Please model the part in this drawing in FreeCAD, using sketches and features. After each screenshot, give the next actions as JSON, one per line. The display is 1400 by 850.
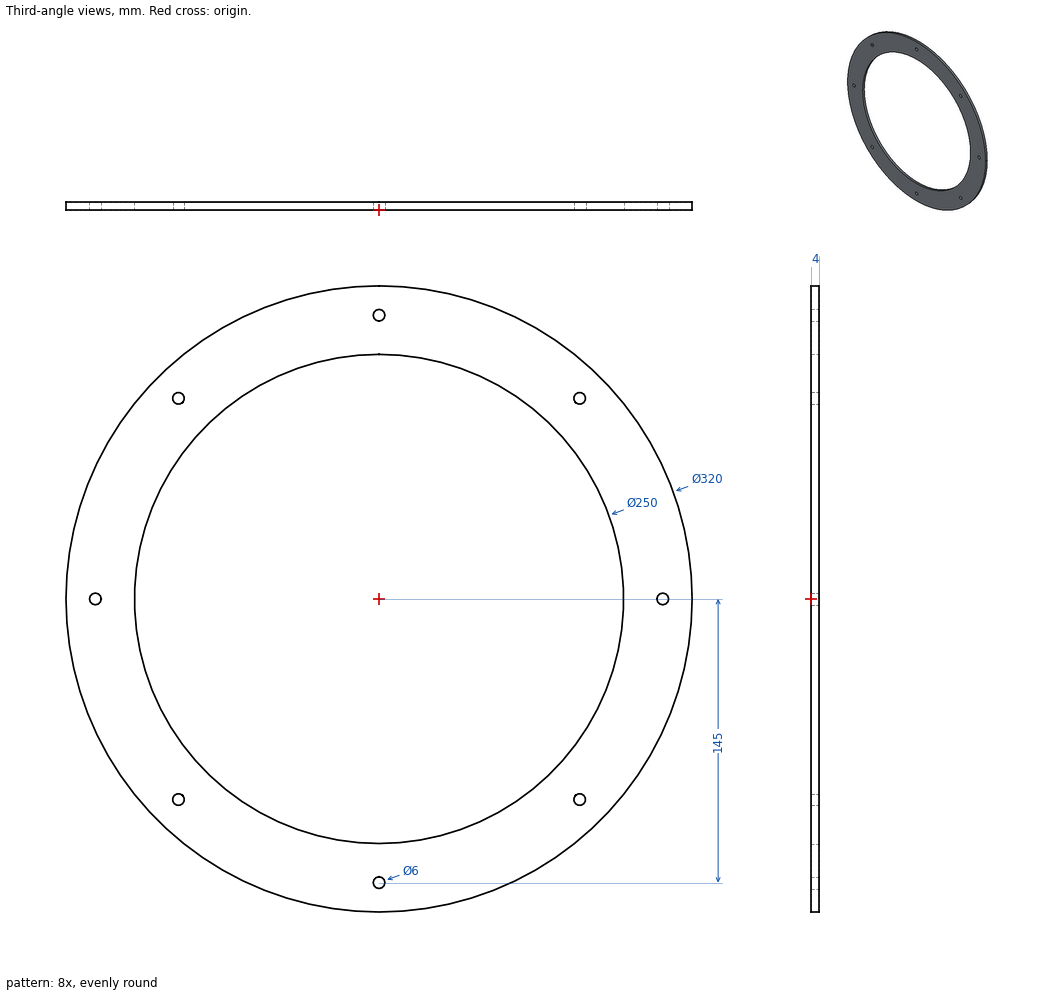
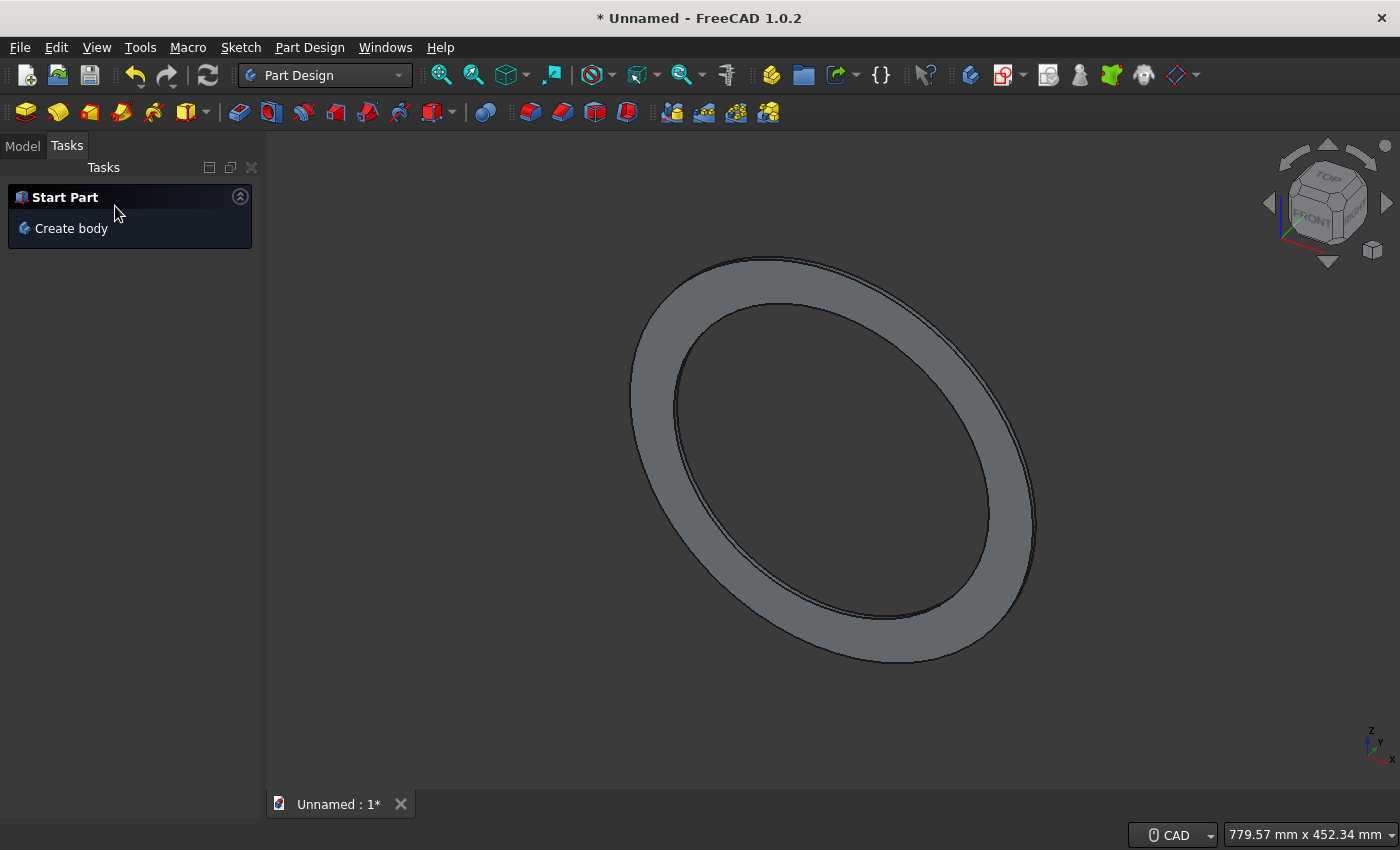
{"action": "key", "text": "4"}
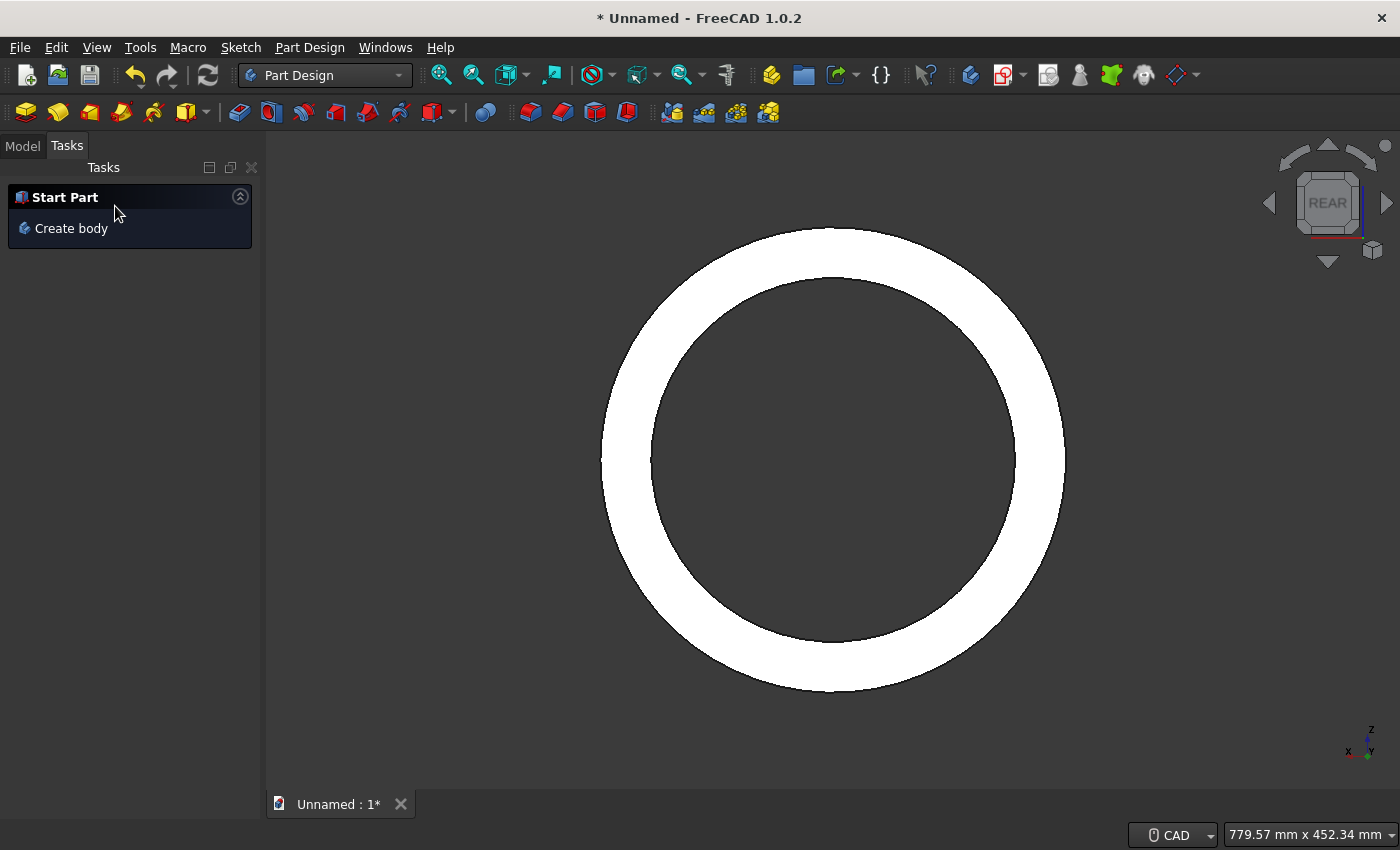
{"action": "left_click", "coordinate": [900, 658]}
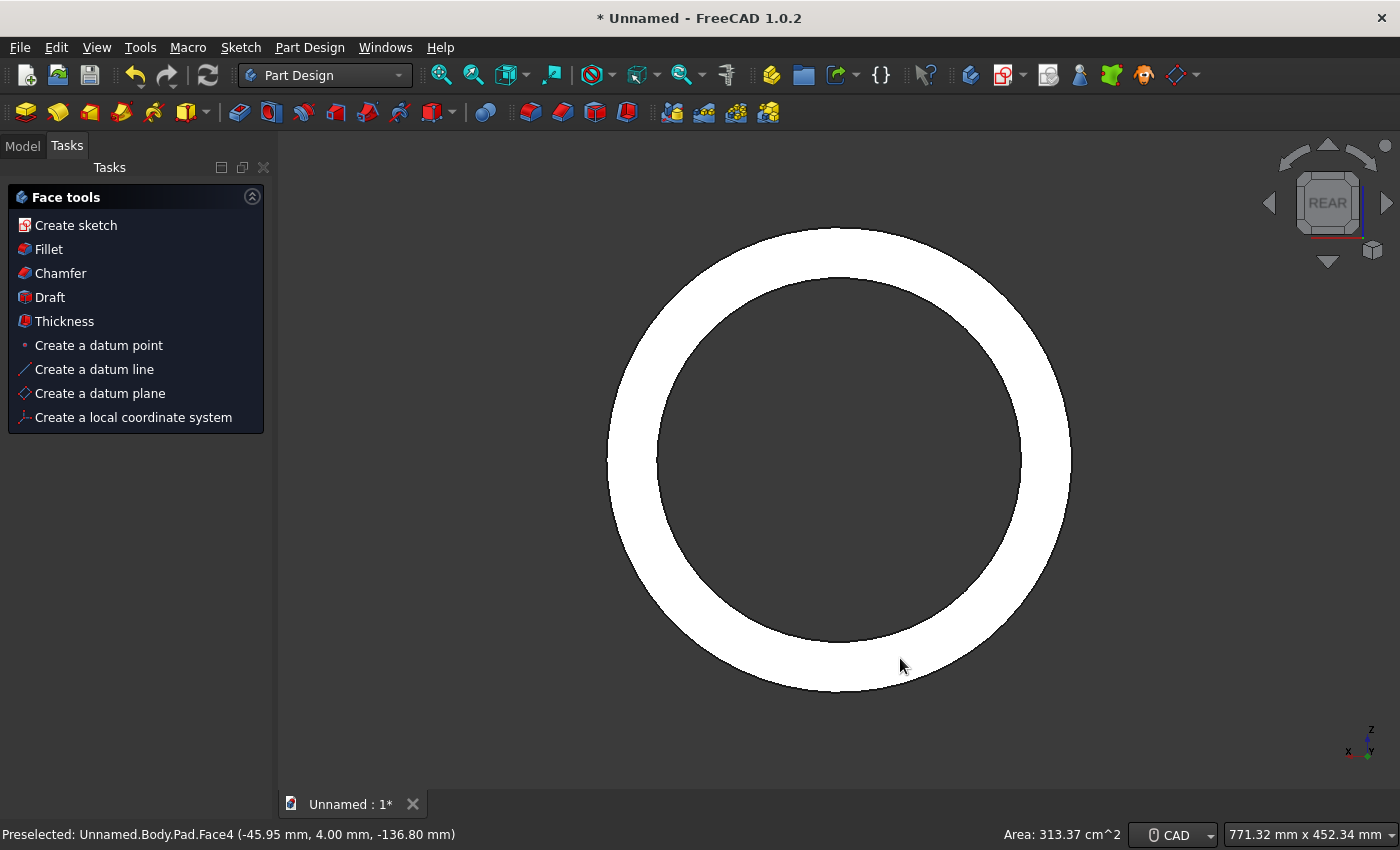
{"action": "left_click", "coordinate": [1004, 76]}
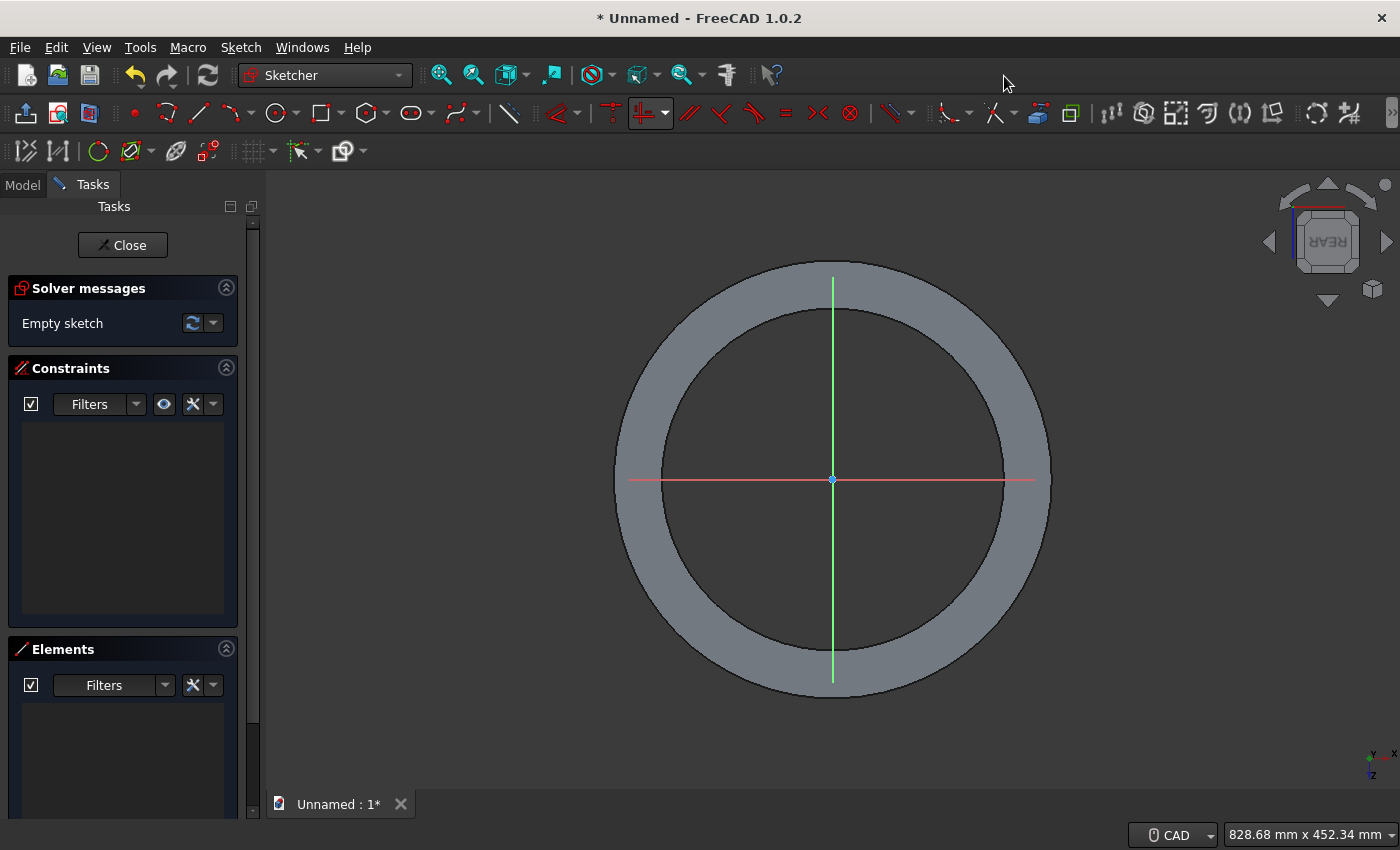
{"action": "scroll", "coordinate": [836, 271], "scroll_direction": "up", "scroll_amount": 15}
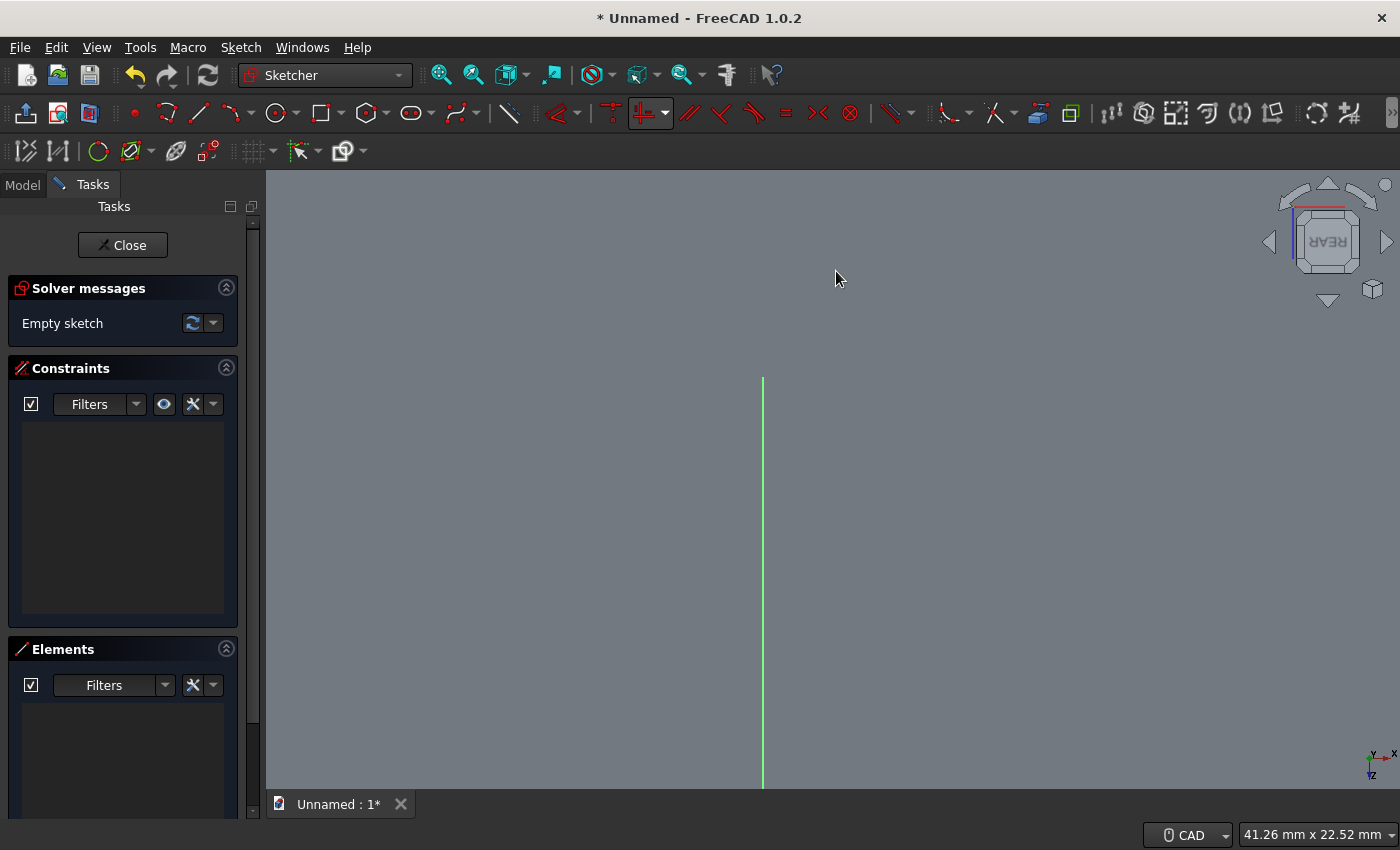
{"action": "scroll", "coordinate": [762, 463], "scroll_direction": "up", "scroll_amount": 4}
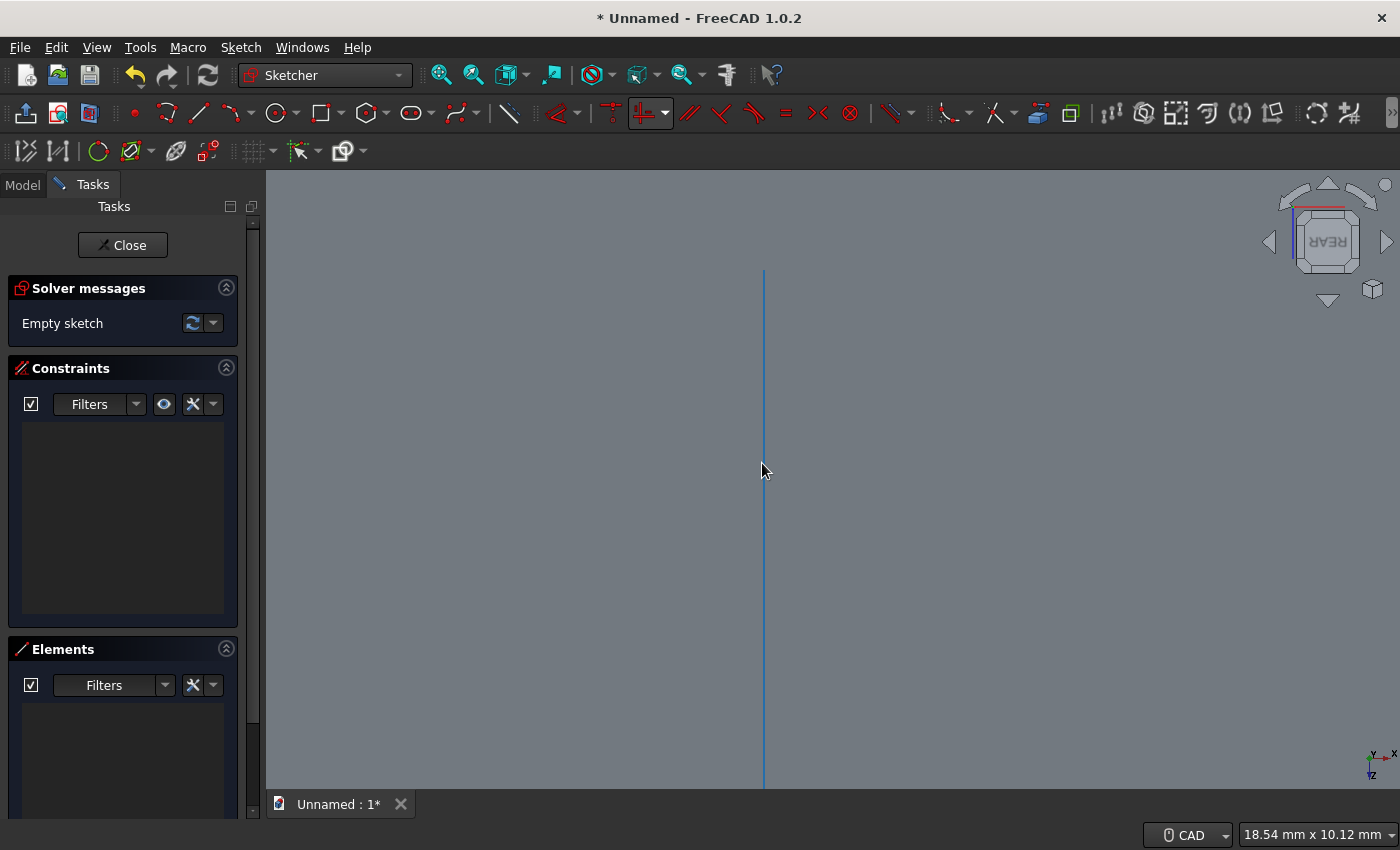
{"action": "key", "text": "g c"}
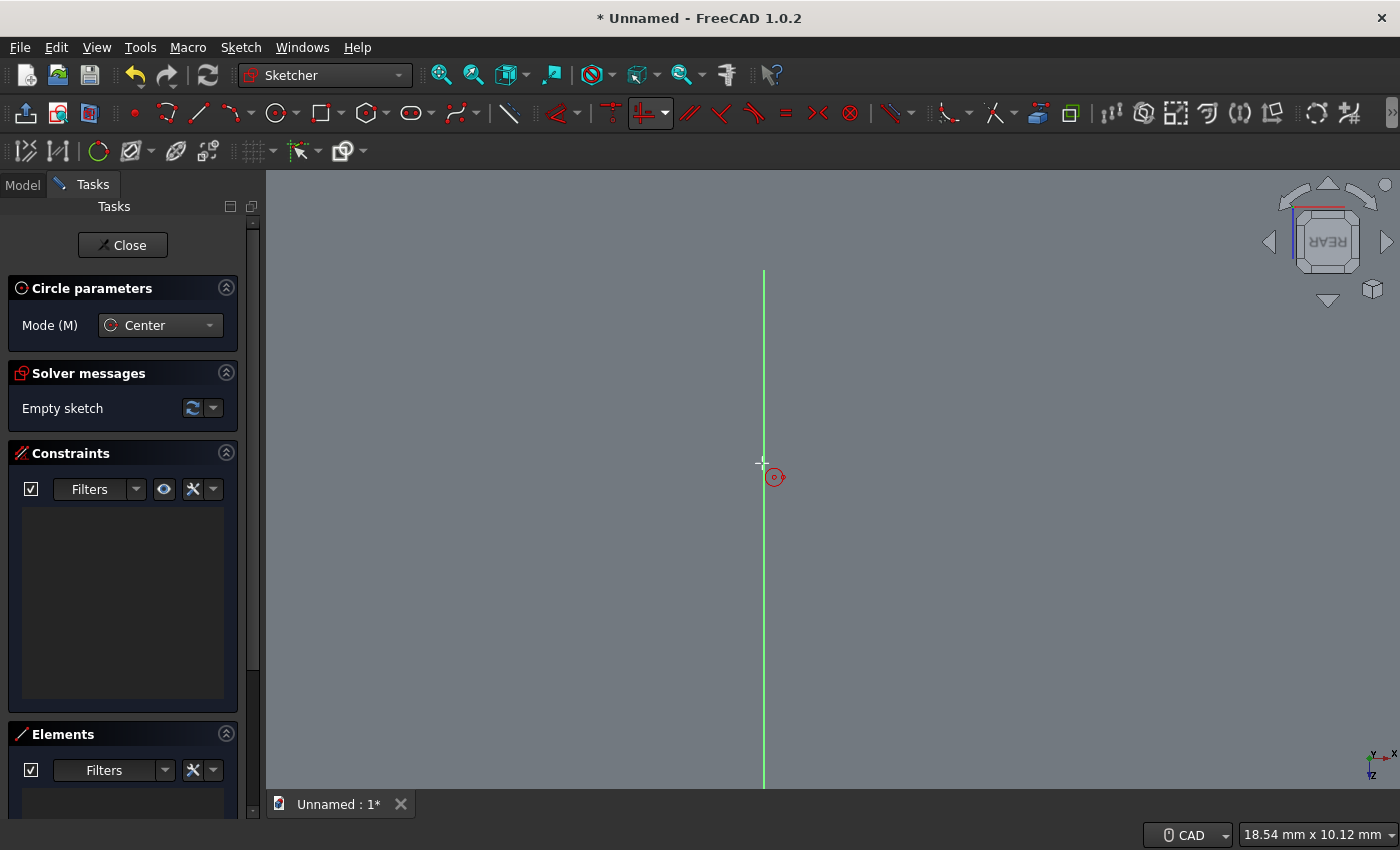
{"action": "left_click", "coordinate": [764, 479]}
{"action": "mouse_move", "coordinate": [894, 349]}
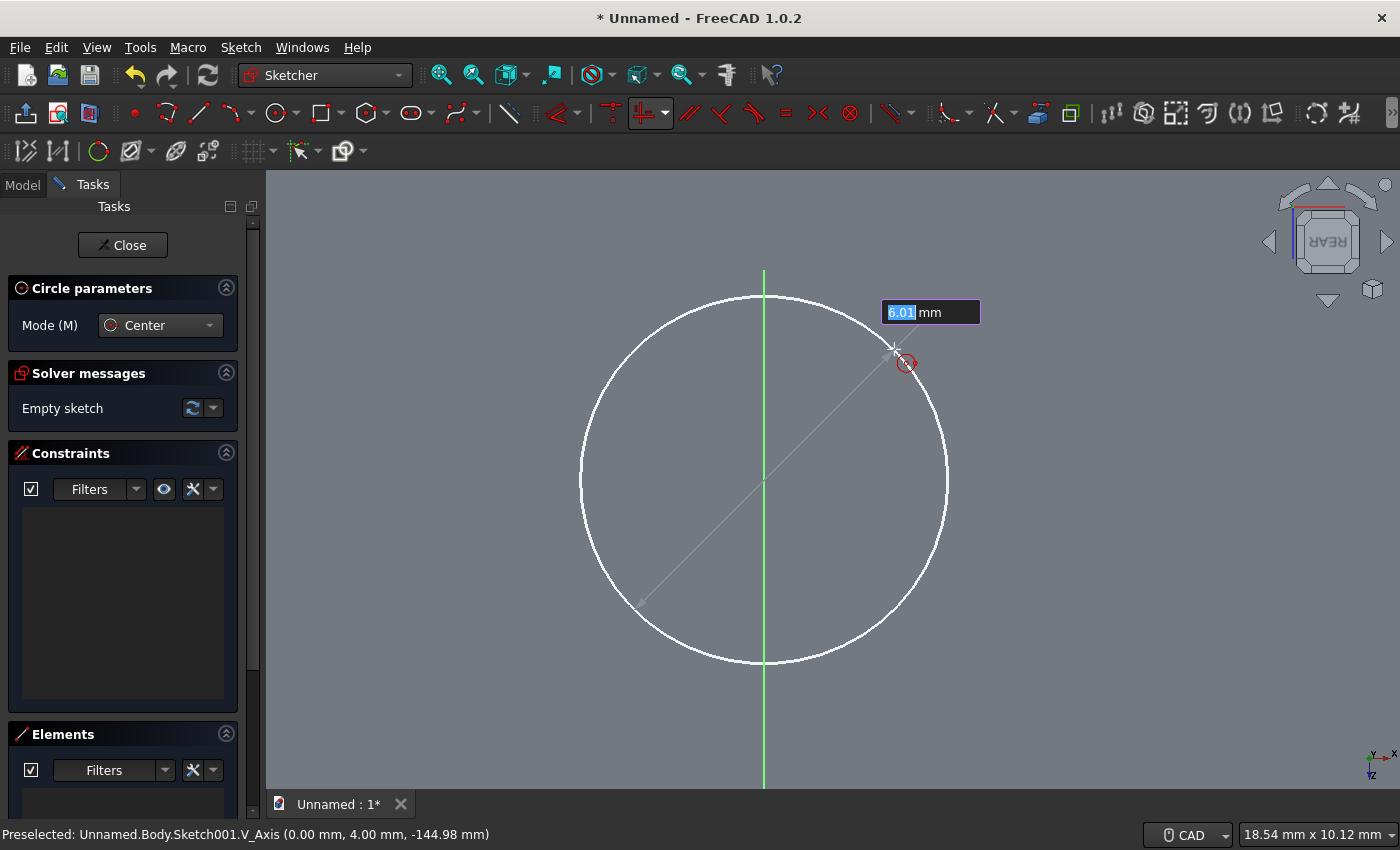
{"action": "type", "text": "6"}
{"action": "key", "text": "Return"}
{"action": "key", "text": "Escape"}